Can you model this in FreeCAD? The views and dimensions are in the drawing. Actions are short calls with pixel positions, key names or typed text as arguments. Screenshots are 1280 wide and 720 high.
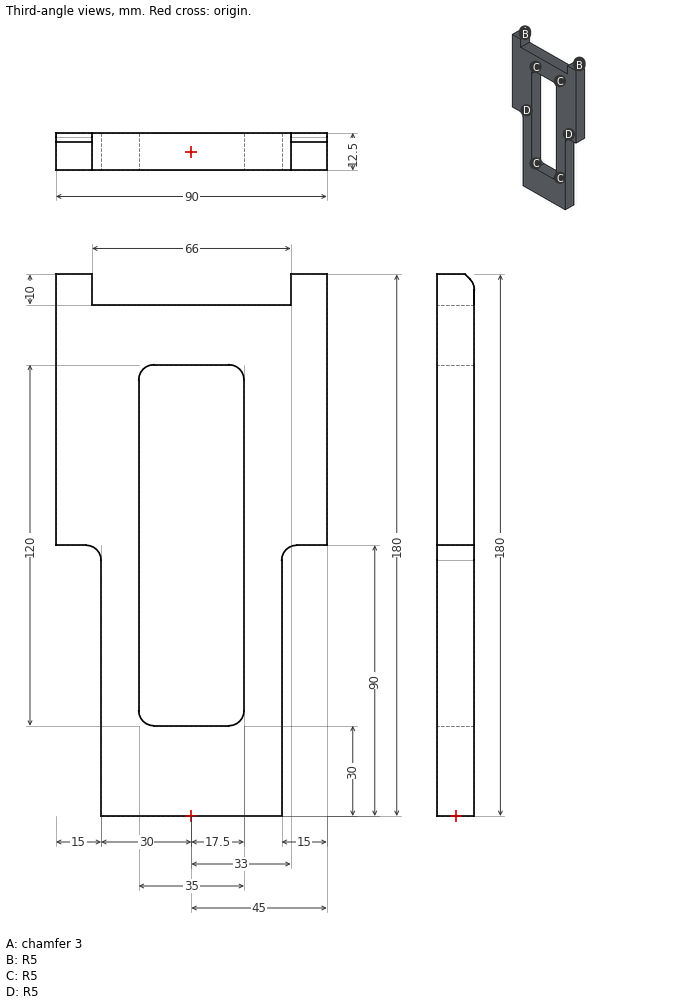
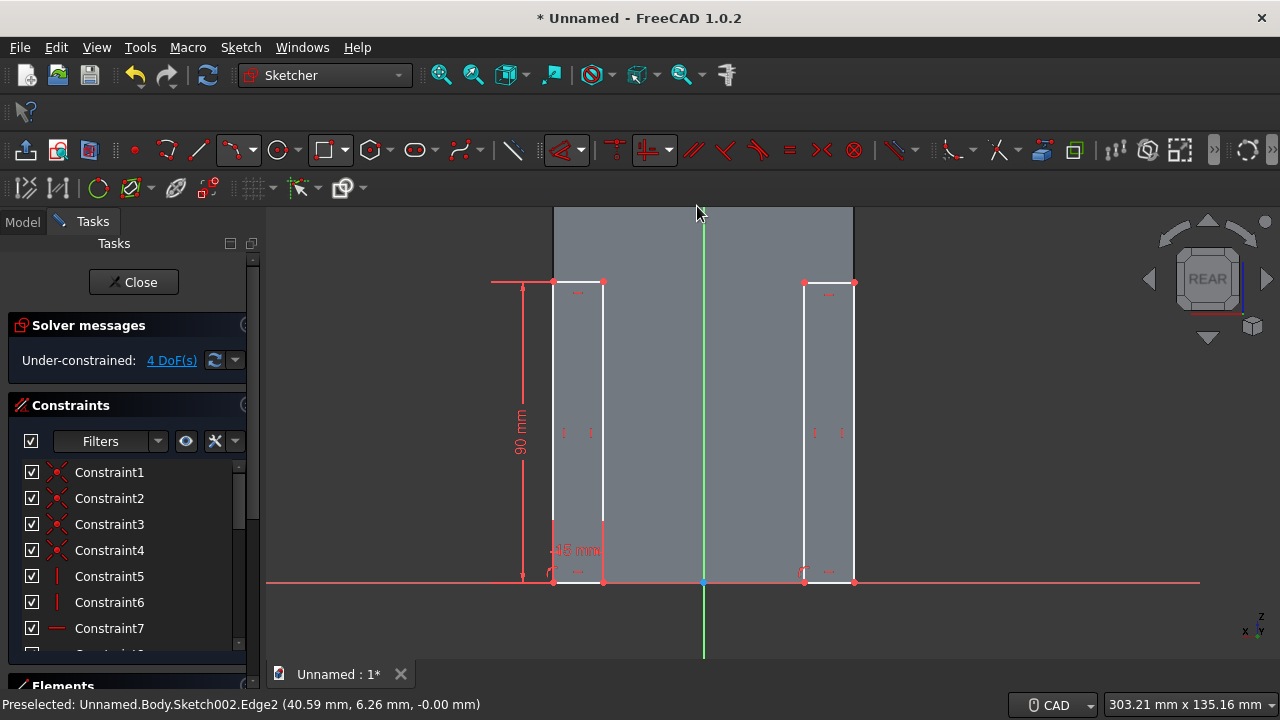
click(804, 373)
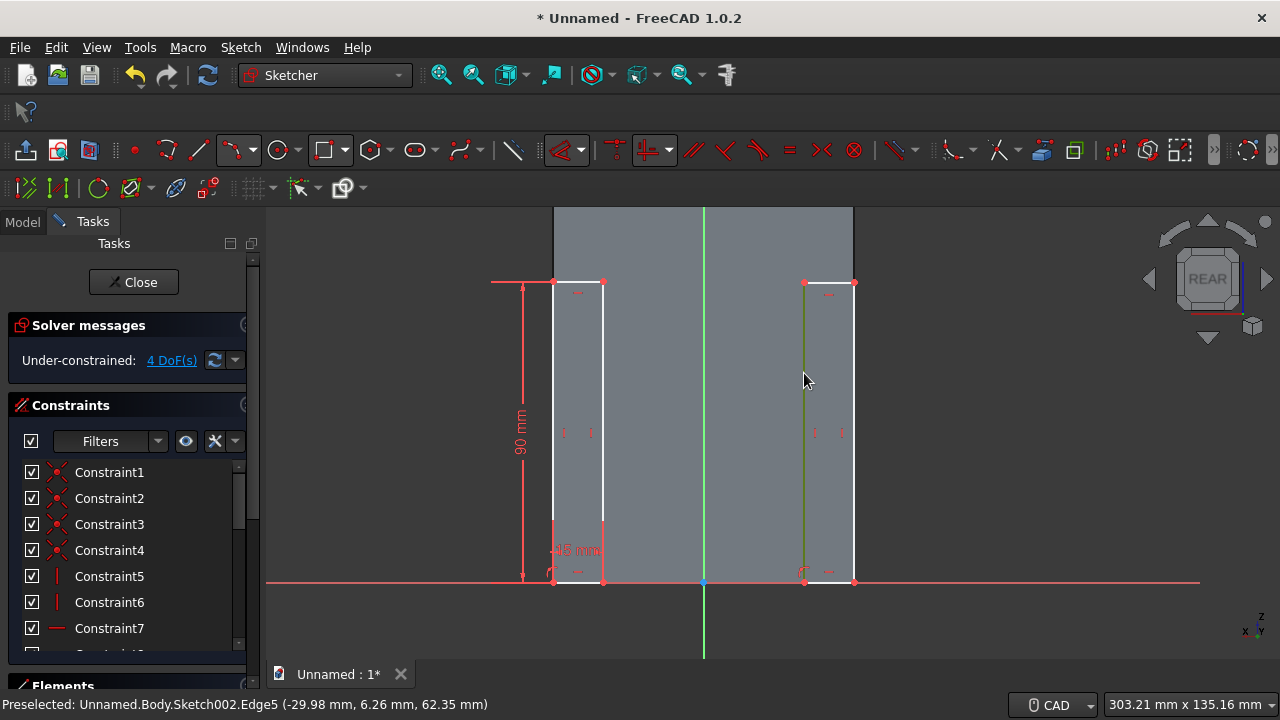
click(584, 150)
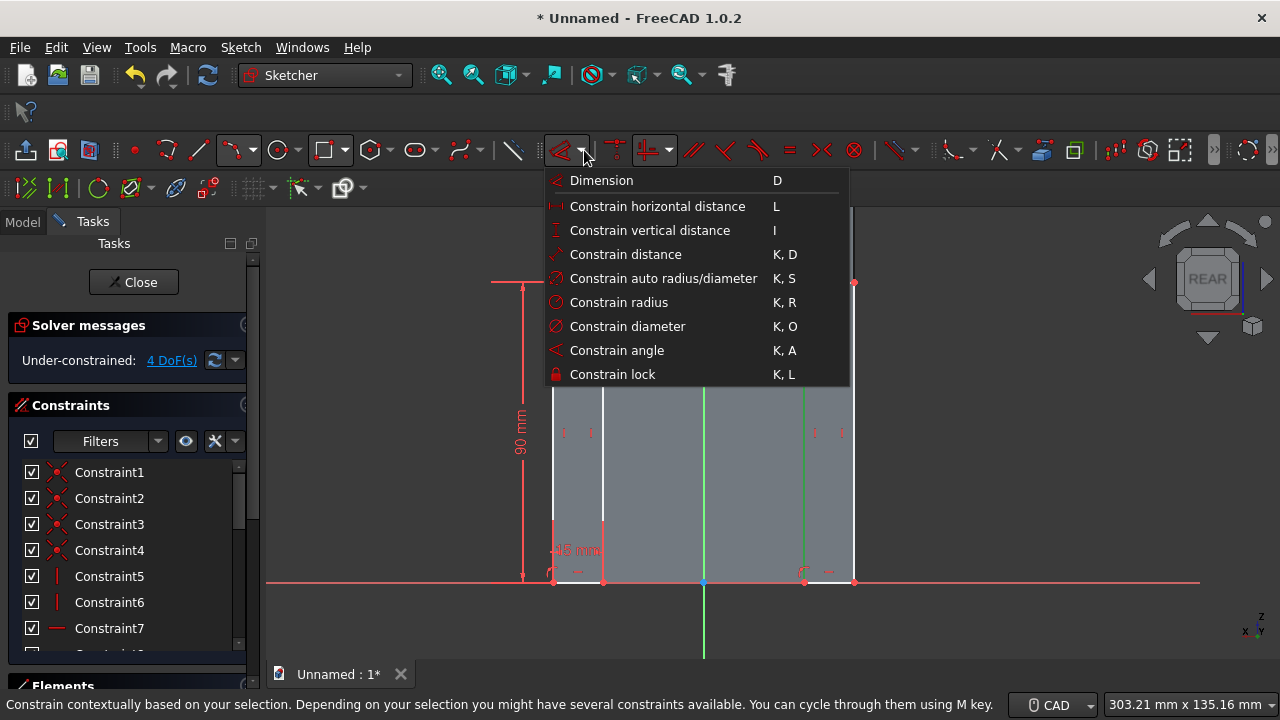
click(697, 230)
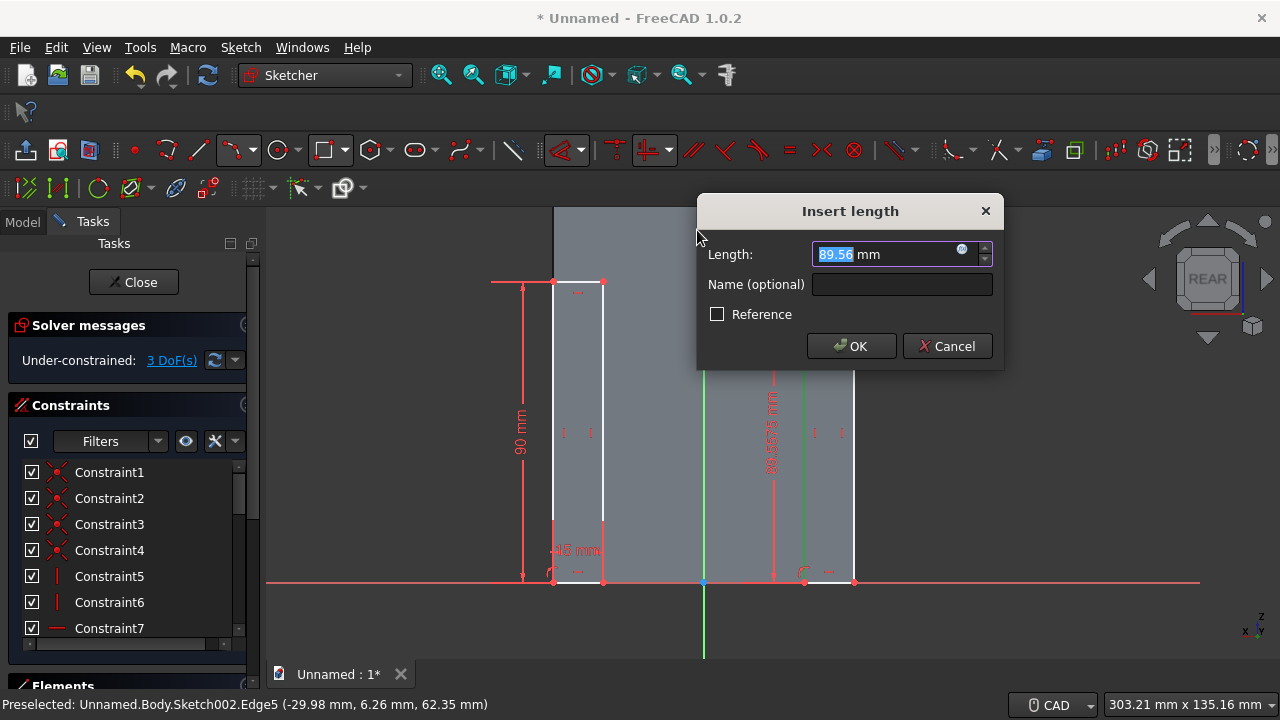
text(90)
key(Return)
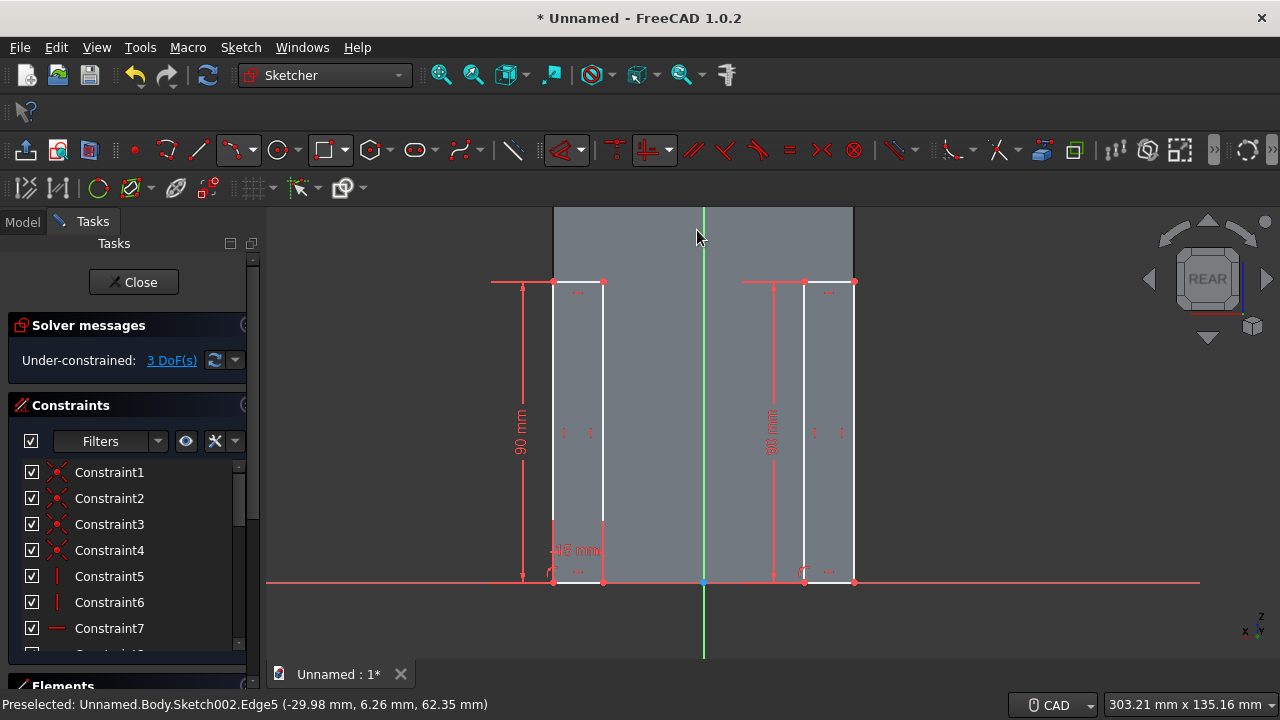
click(819, 582)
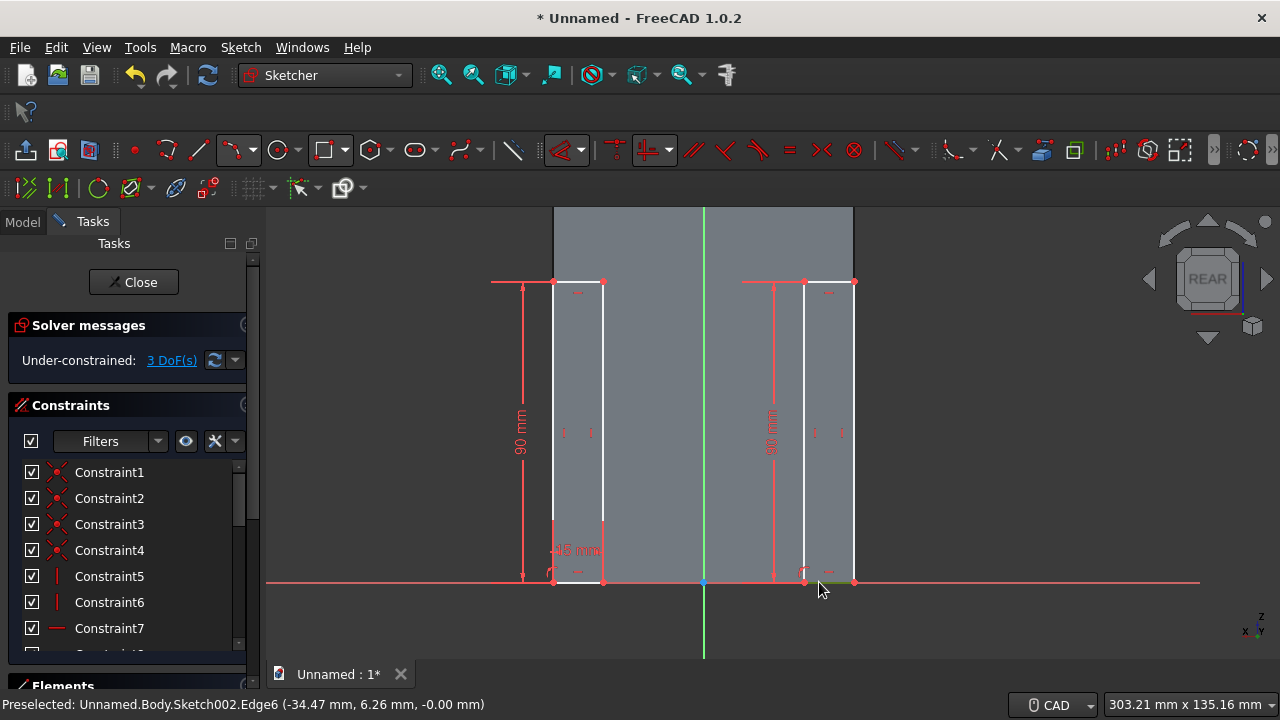
key(l)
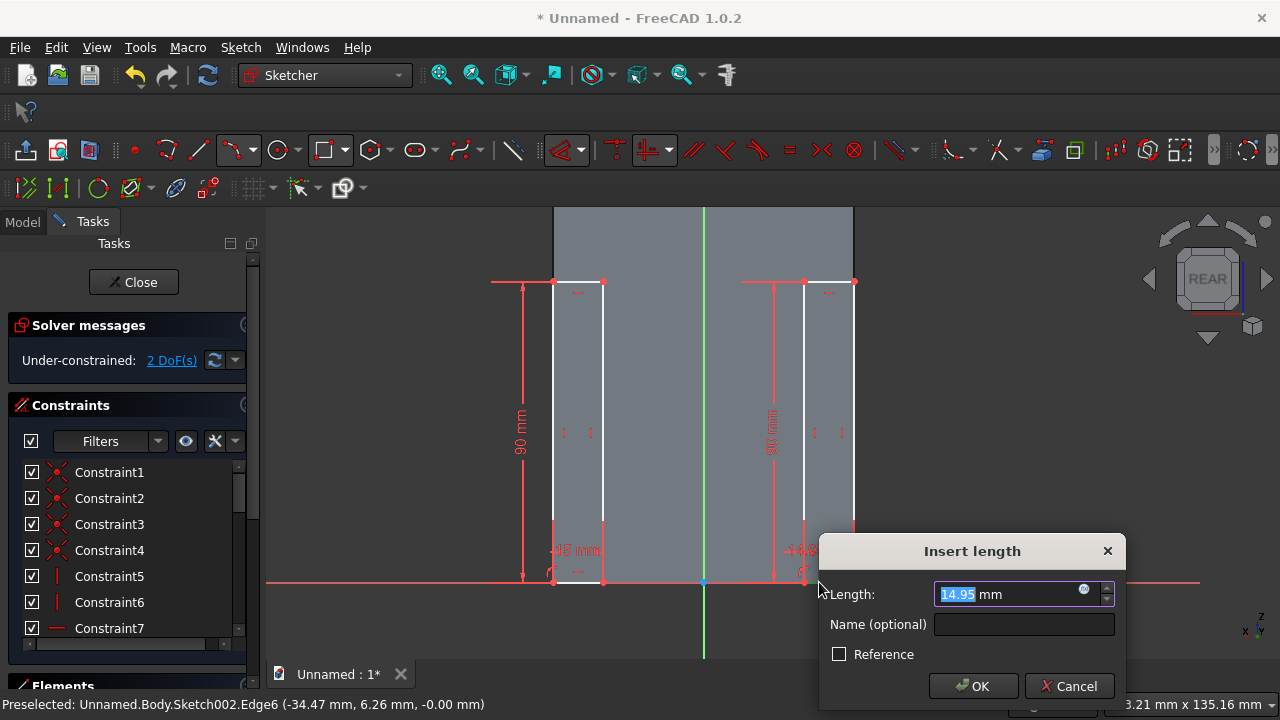
text(15)
key(Return)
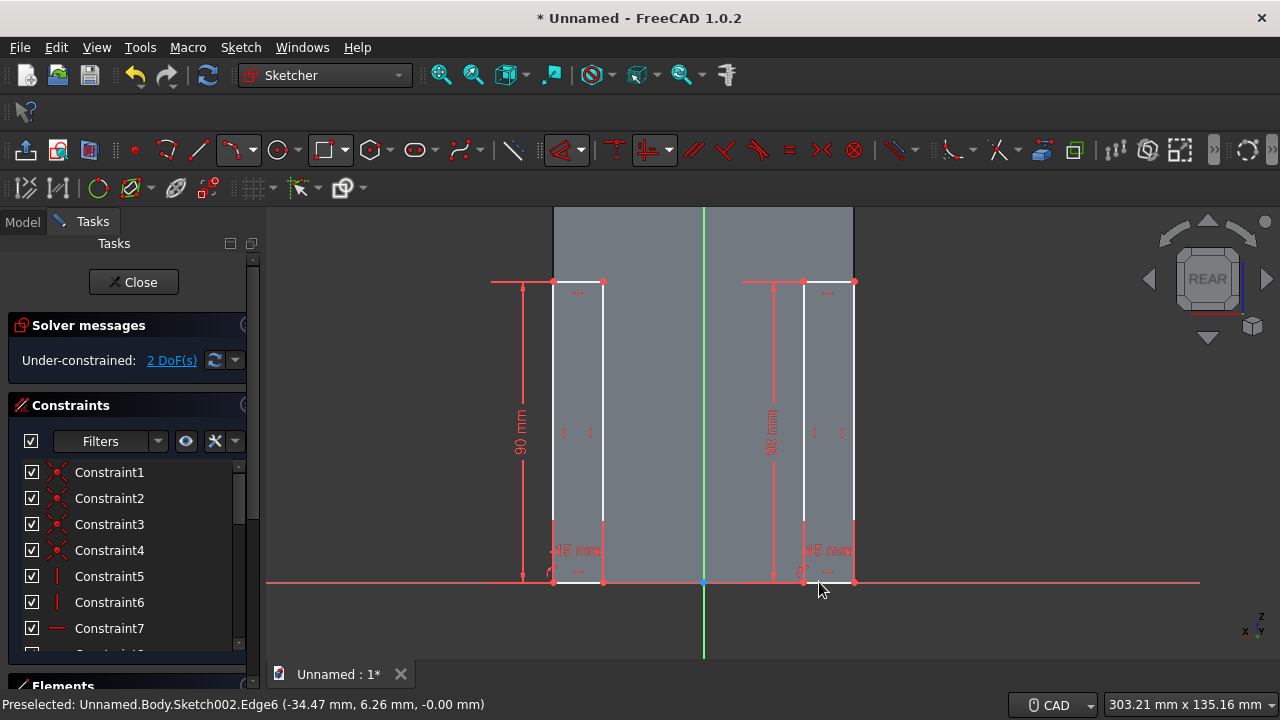
click(553, 282)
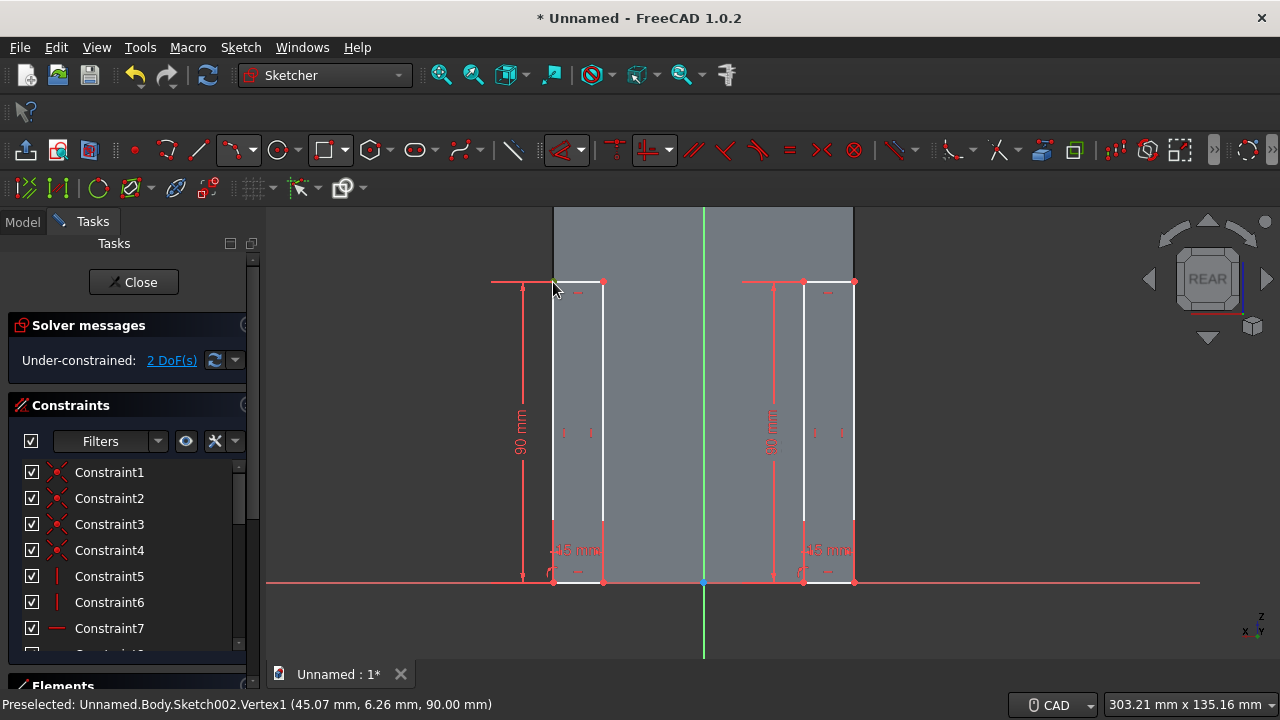
key(l)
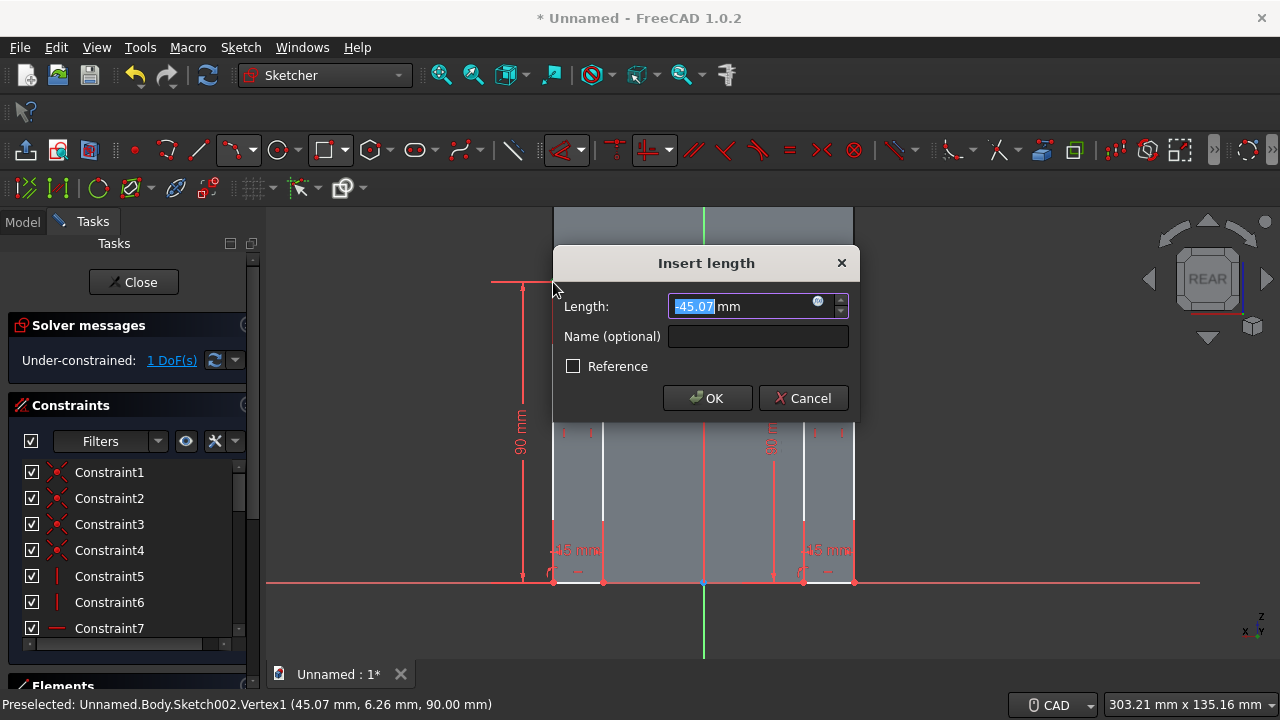
text(-45)
key(Return)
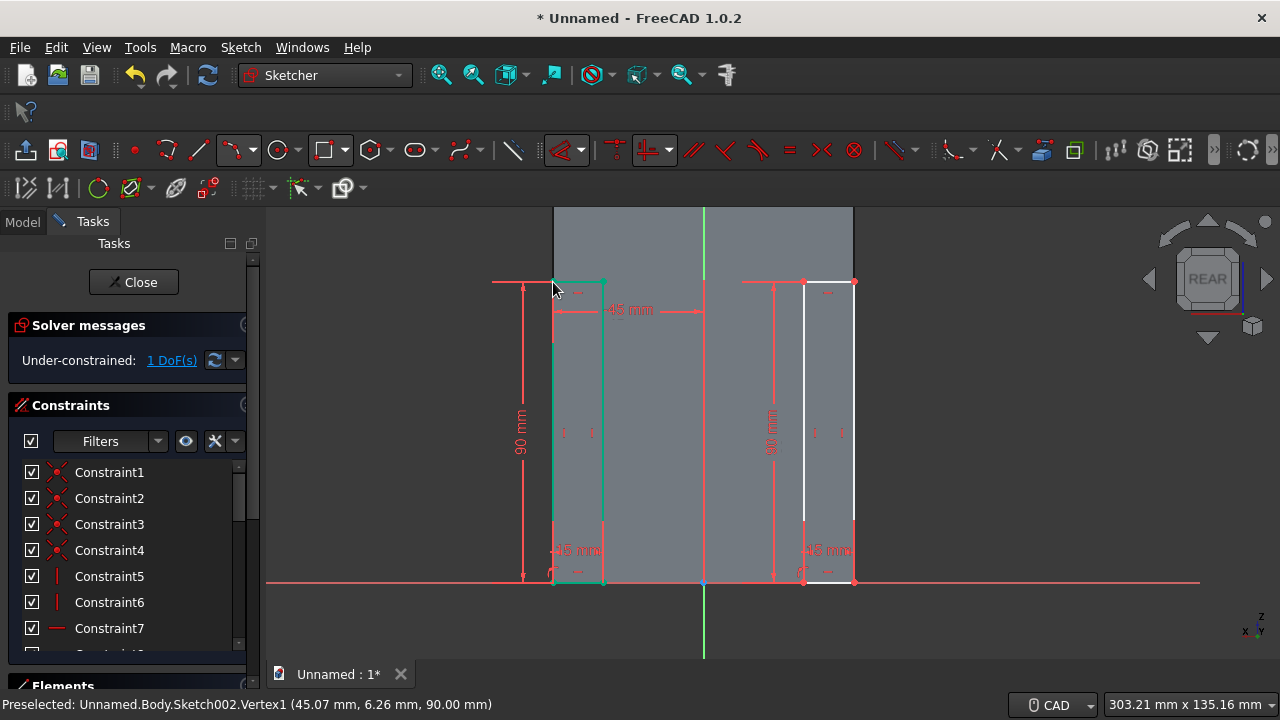
click(804, 282)